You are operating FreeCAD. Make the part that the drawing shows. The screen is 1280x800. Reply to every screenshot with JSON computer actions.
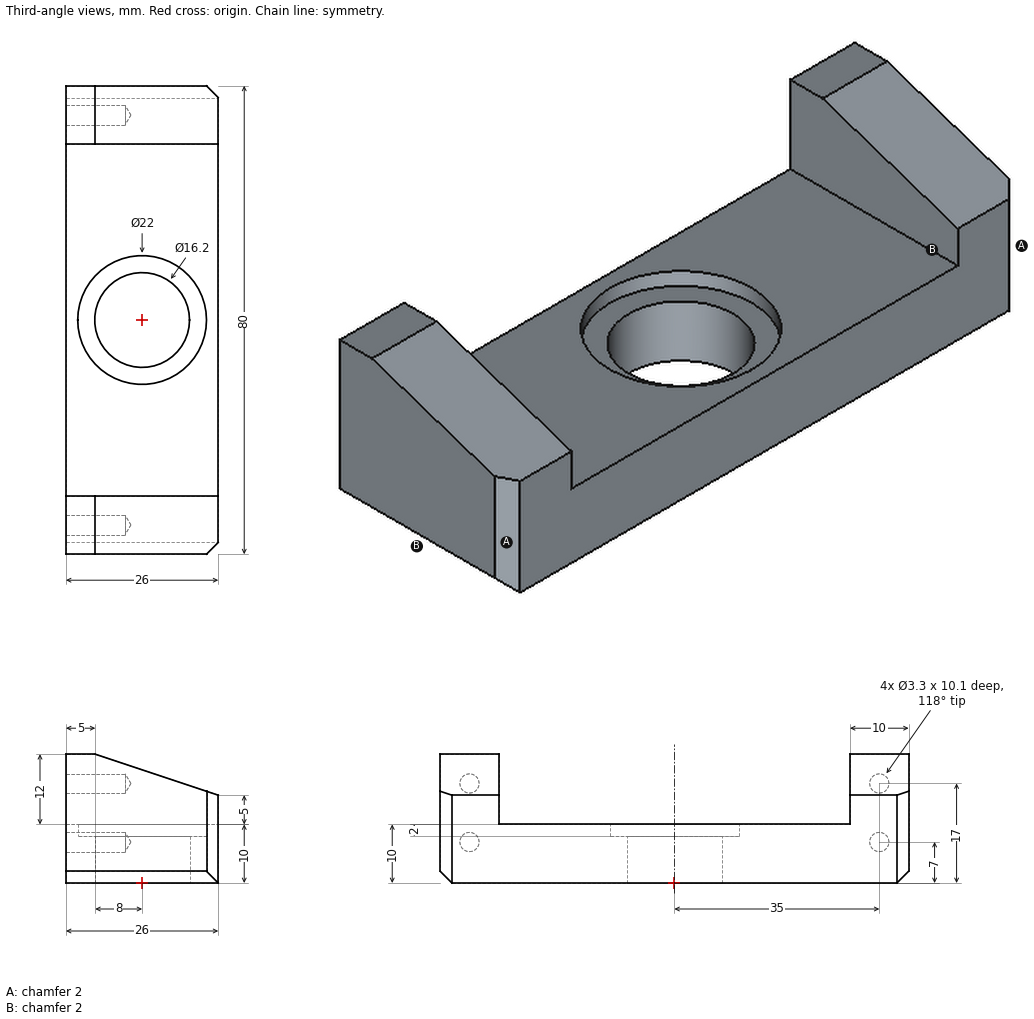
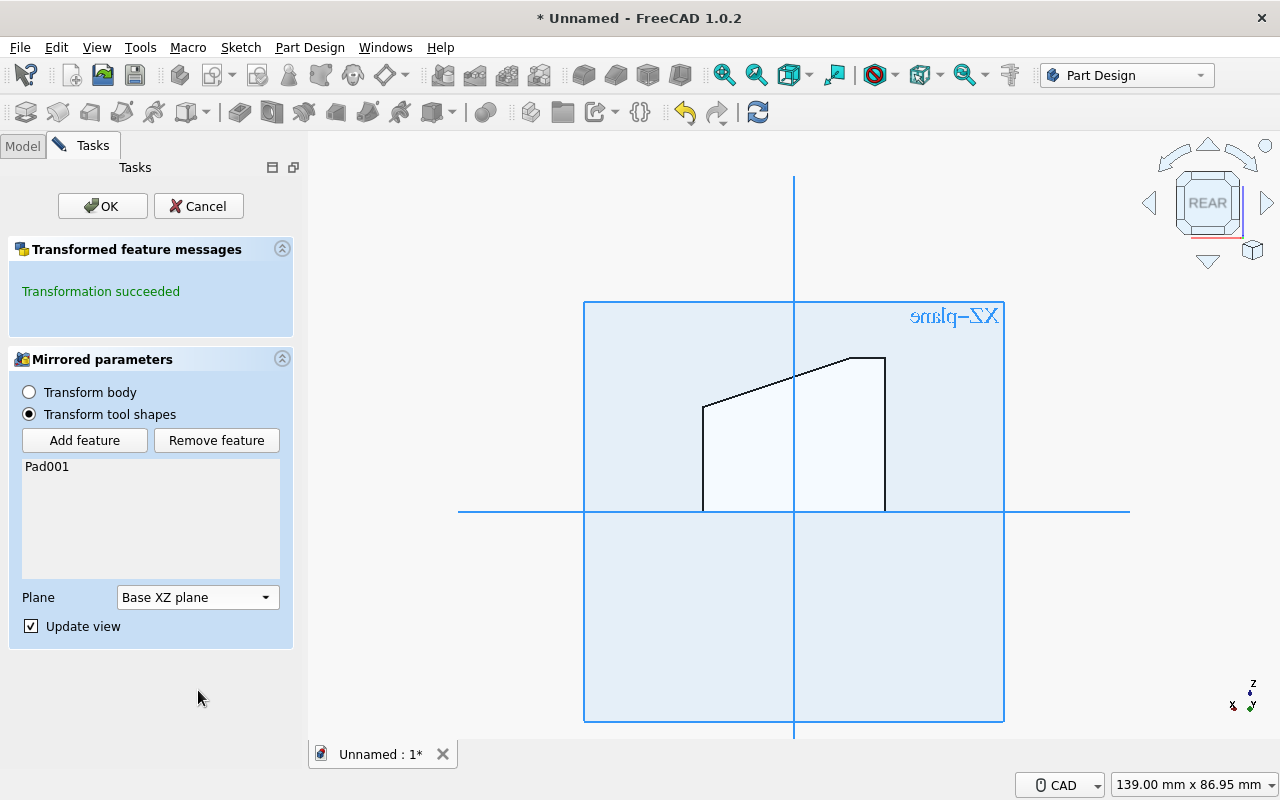
{"action": "left_click", "coordinate": [103, 206]}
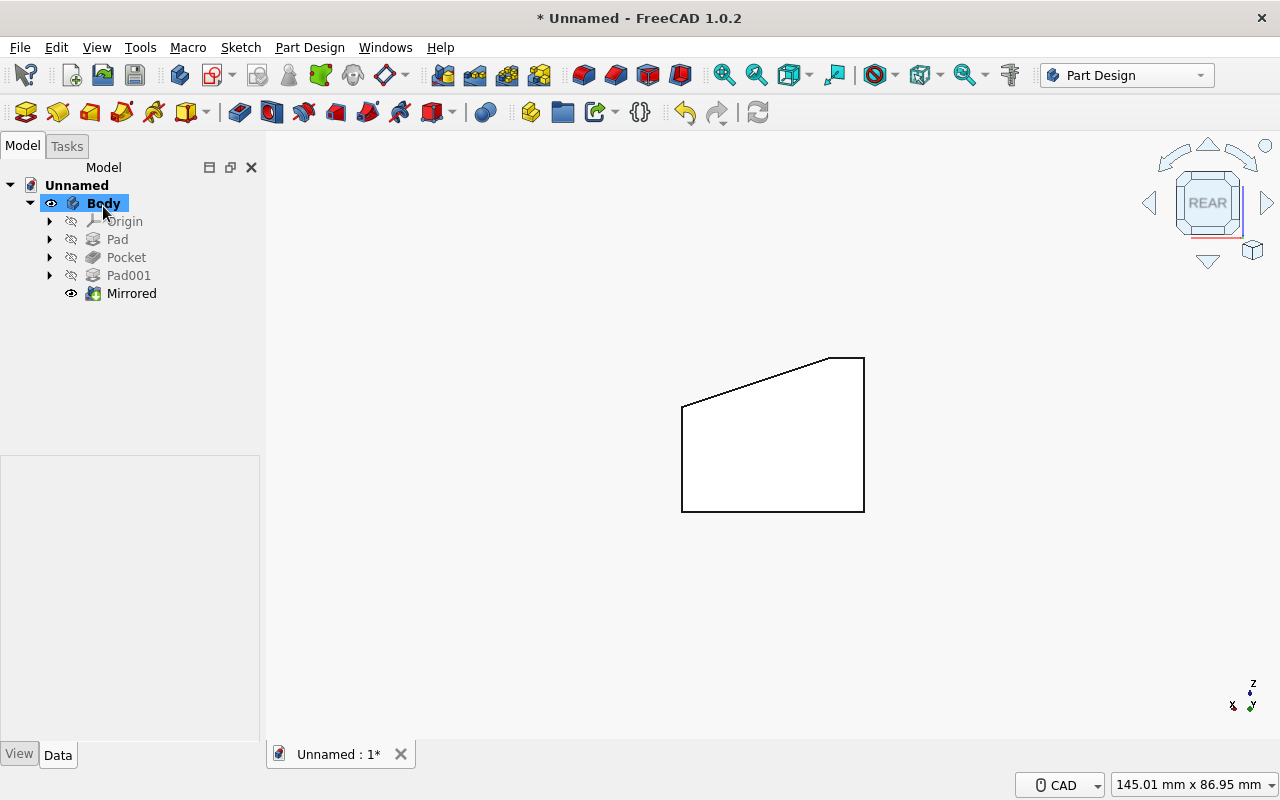
{"action": "left_click", "coordinate": [726, 76]}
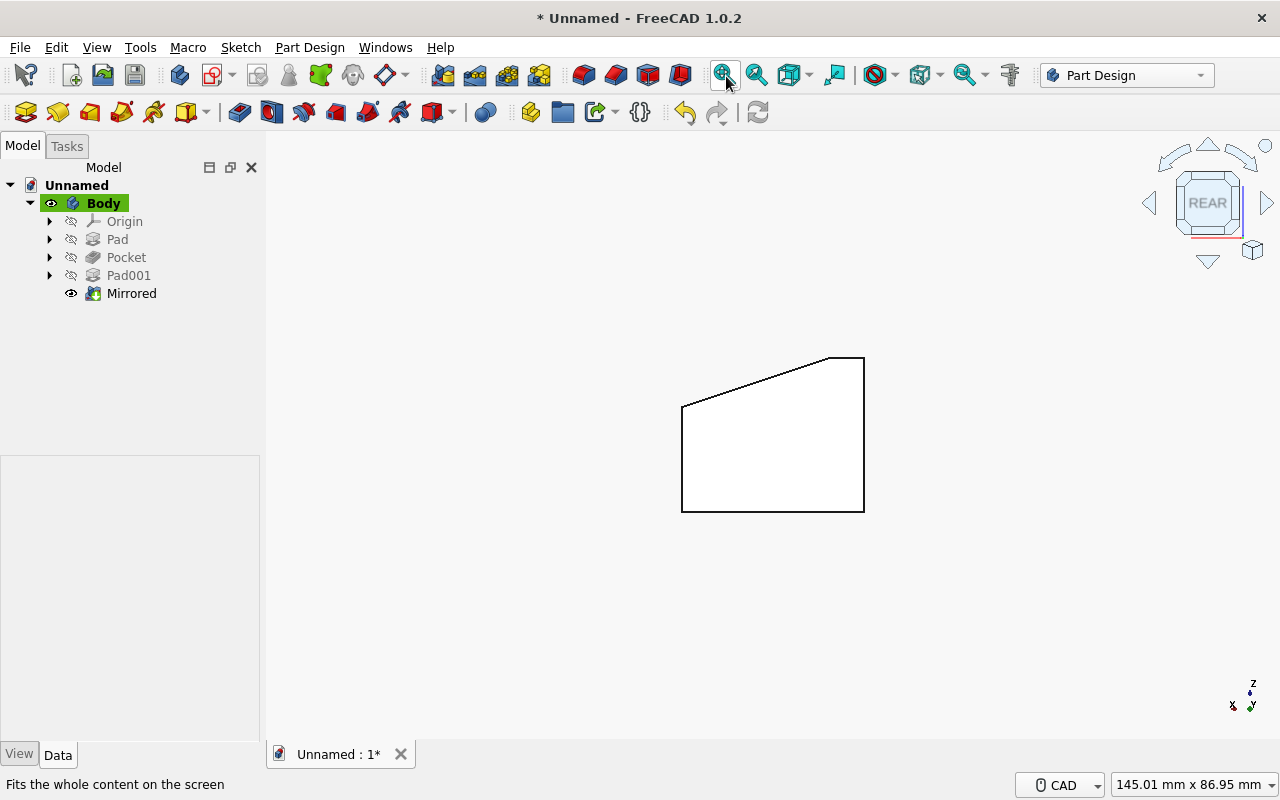
{"action": "key", "text": "0"}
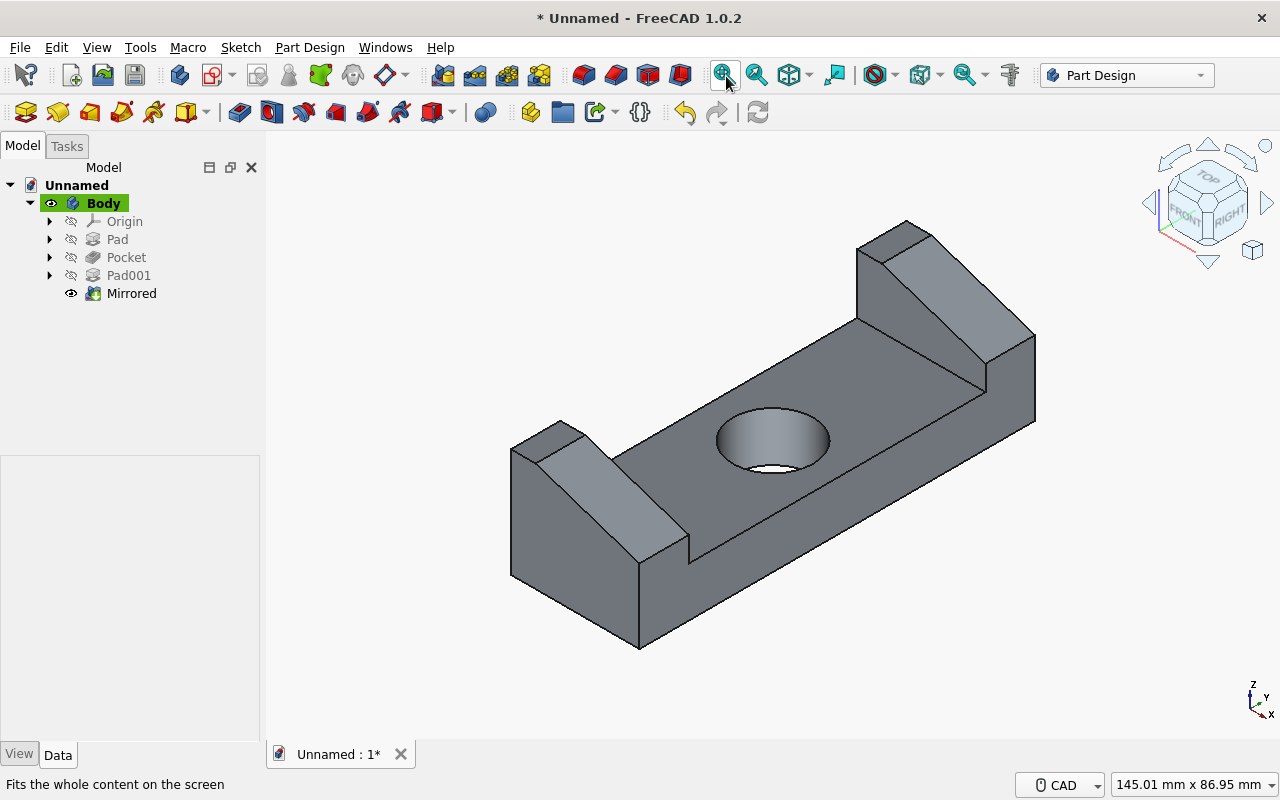
{"action": "left_click", "coordinate": [639, 605]}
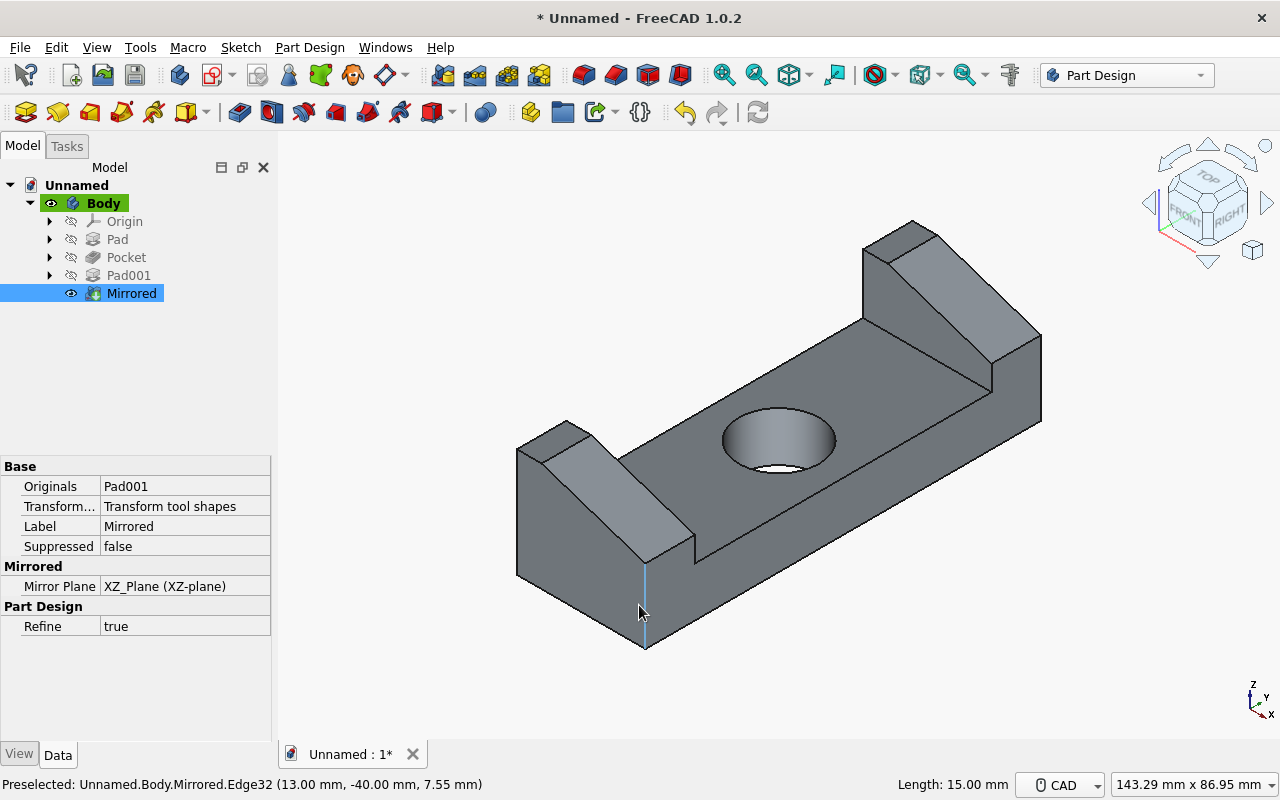
{"action": "key", "text": "2"}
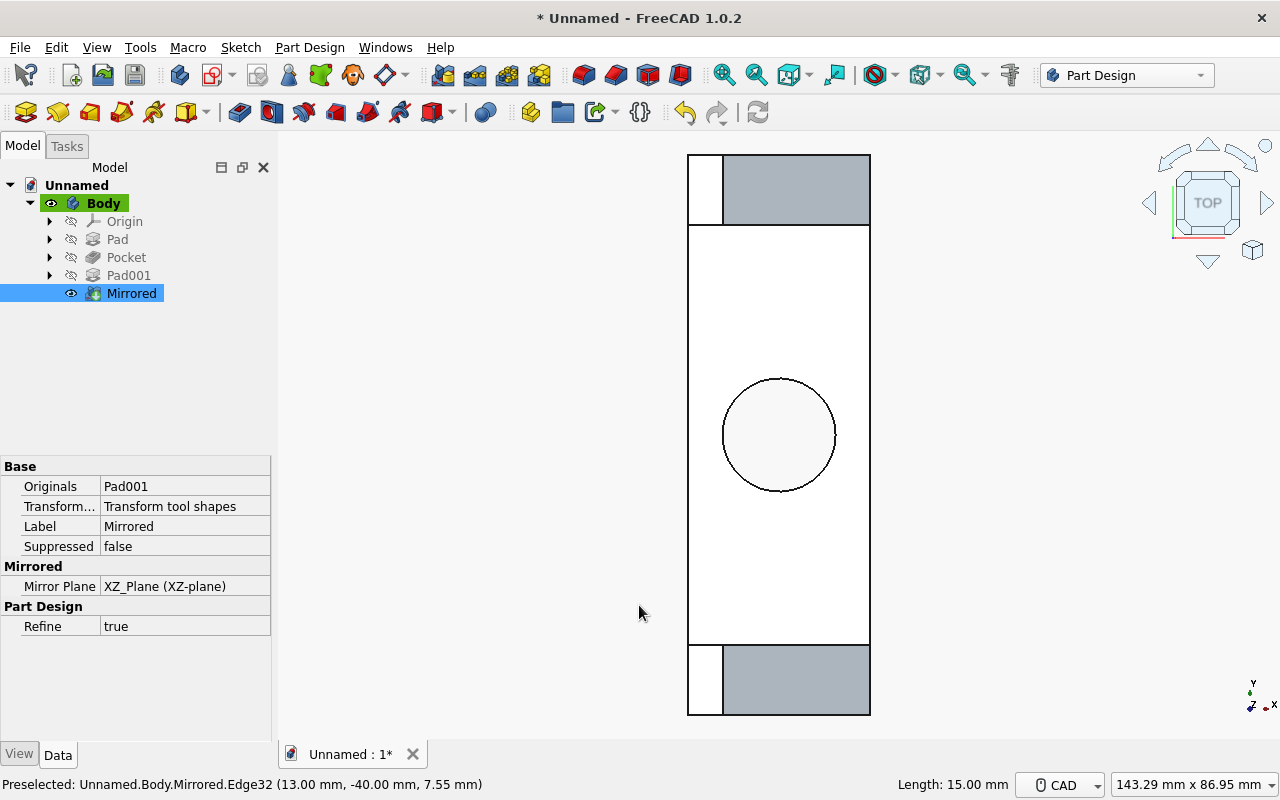
{"action": "key", "text": "1"}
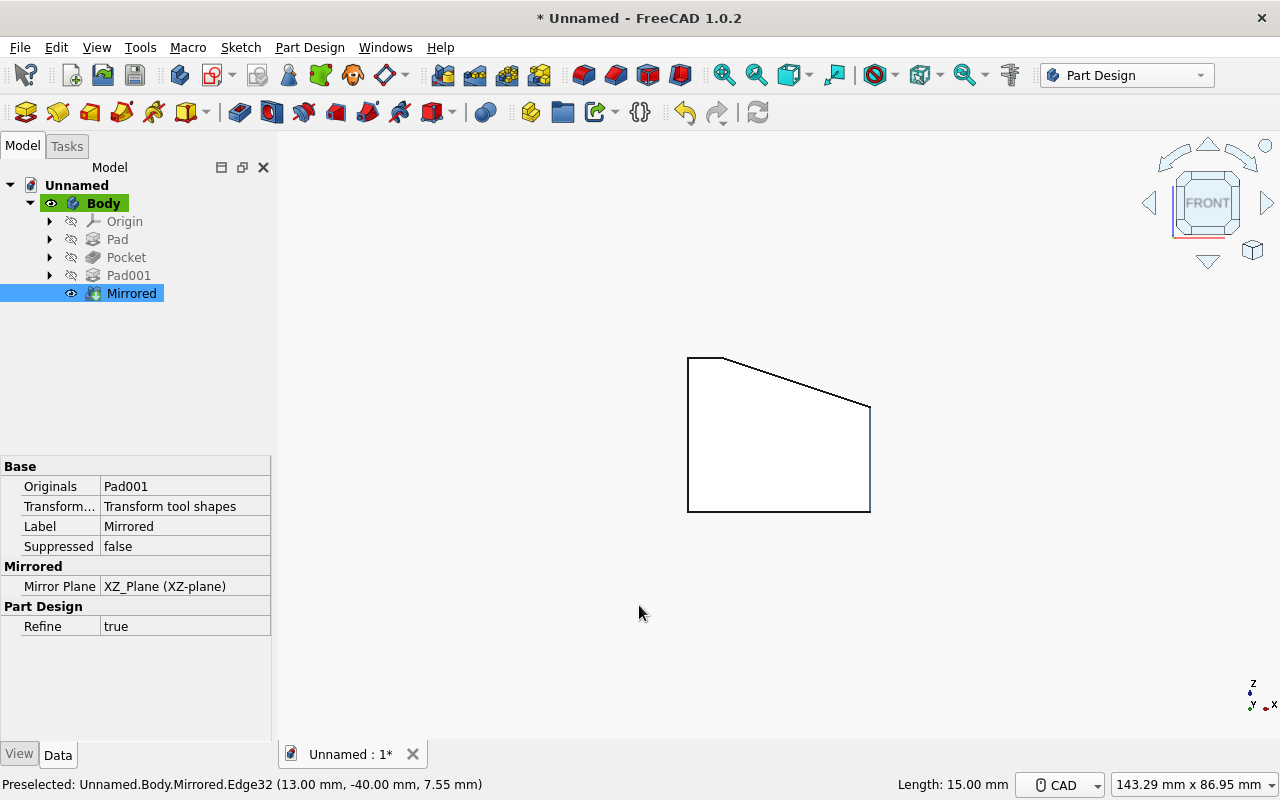
{"action": "left_click", "coordinate": [726, 76]}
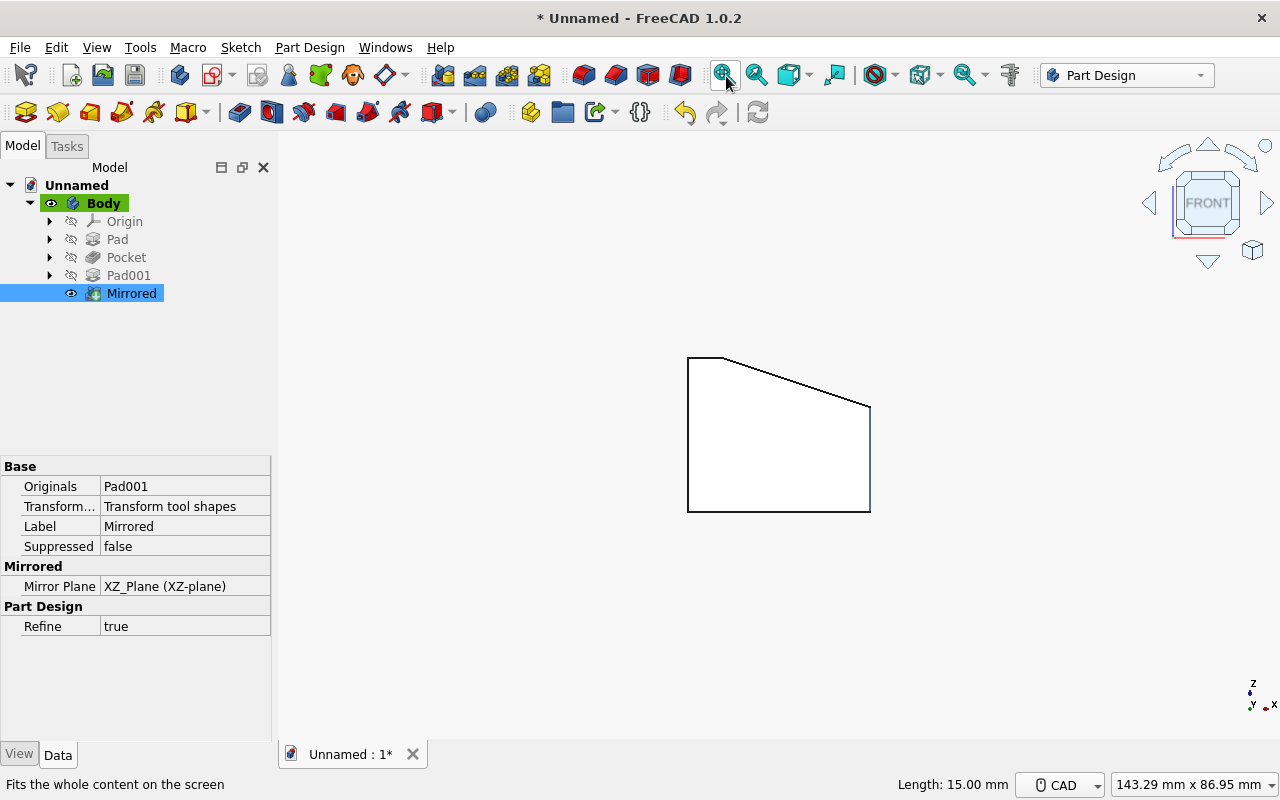
{"action": "key", "text": "3"}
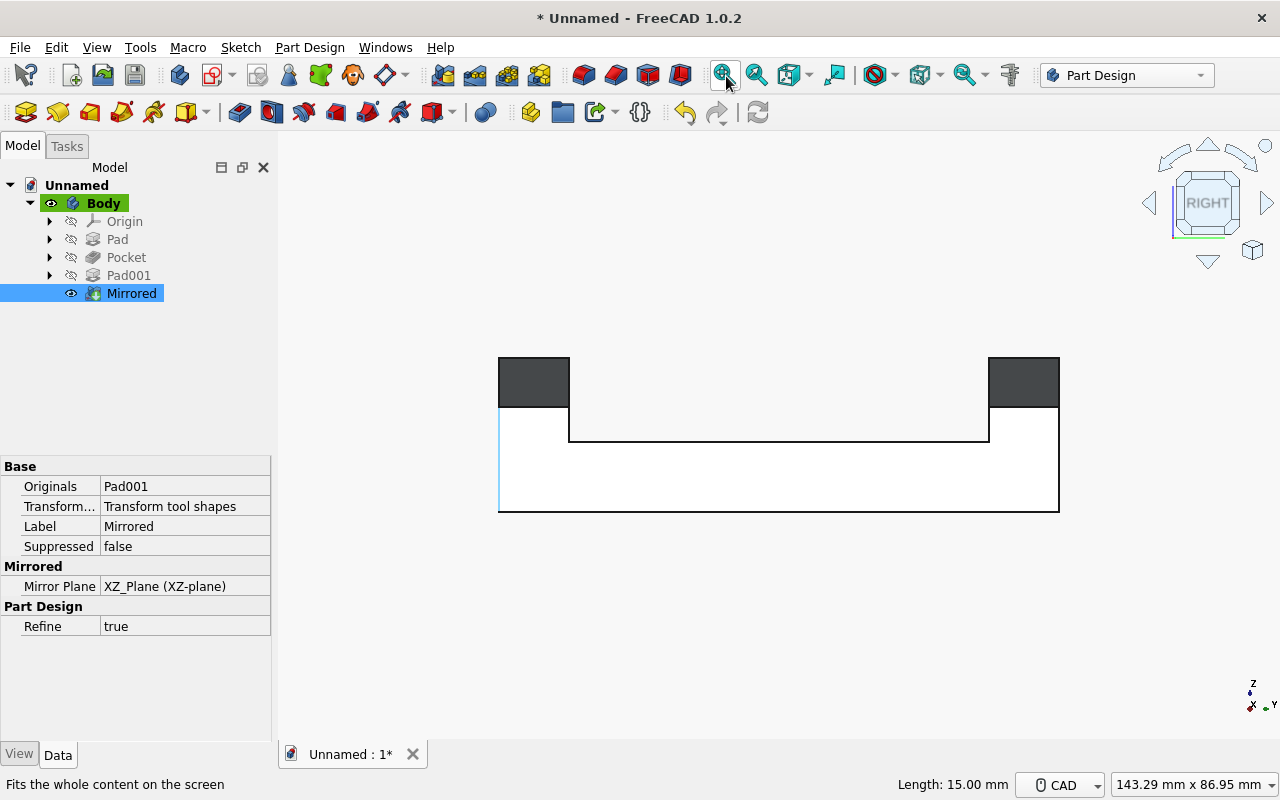
{"action": "left_click", "coordinate": [1059, 458], "text": "ctrl"}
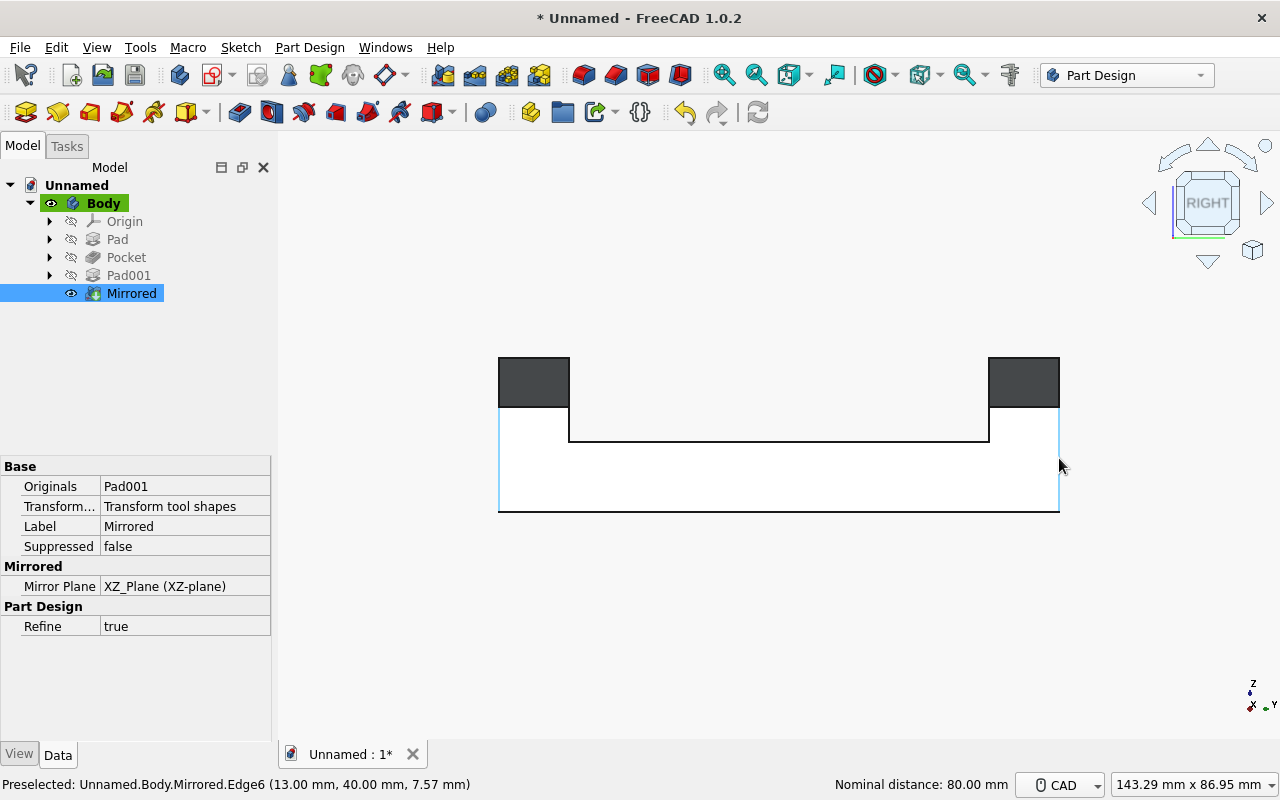
{"action": "left_click", "coordinate": [616, 76]}